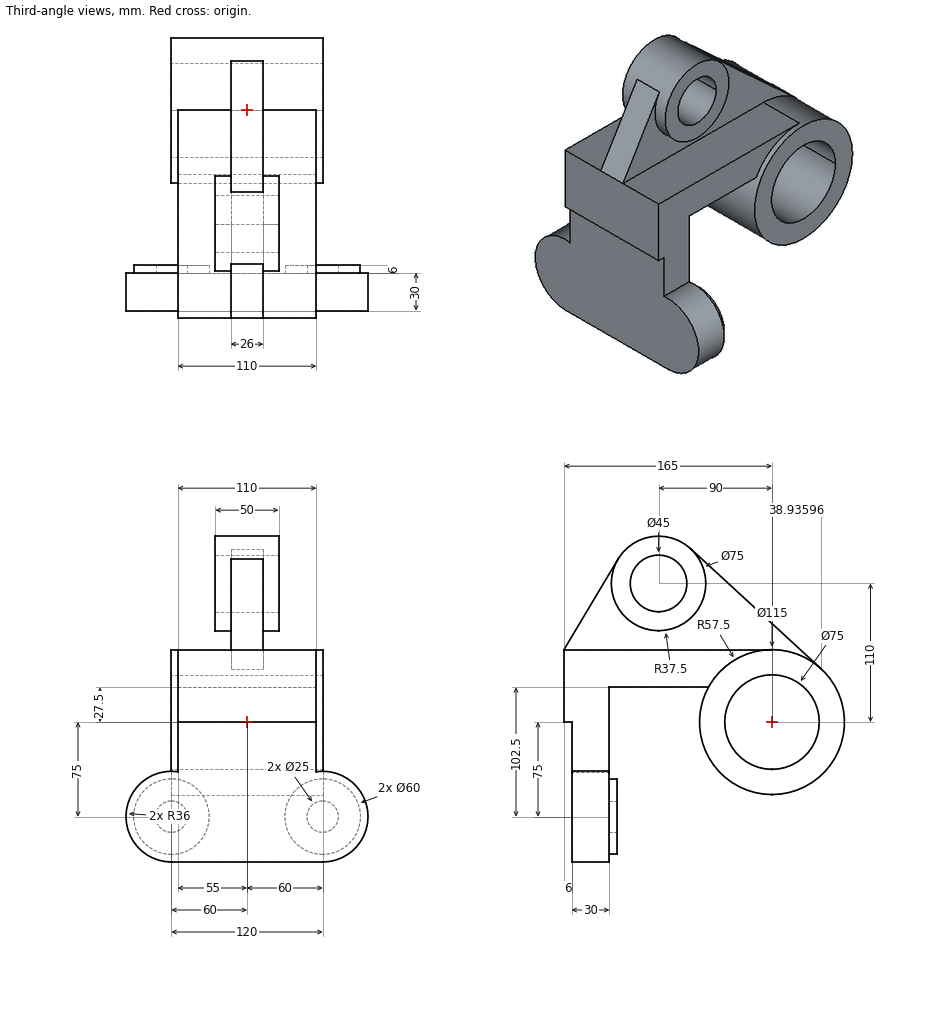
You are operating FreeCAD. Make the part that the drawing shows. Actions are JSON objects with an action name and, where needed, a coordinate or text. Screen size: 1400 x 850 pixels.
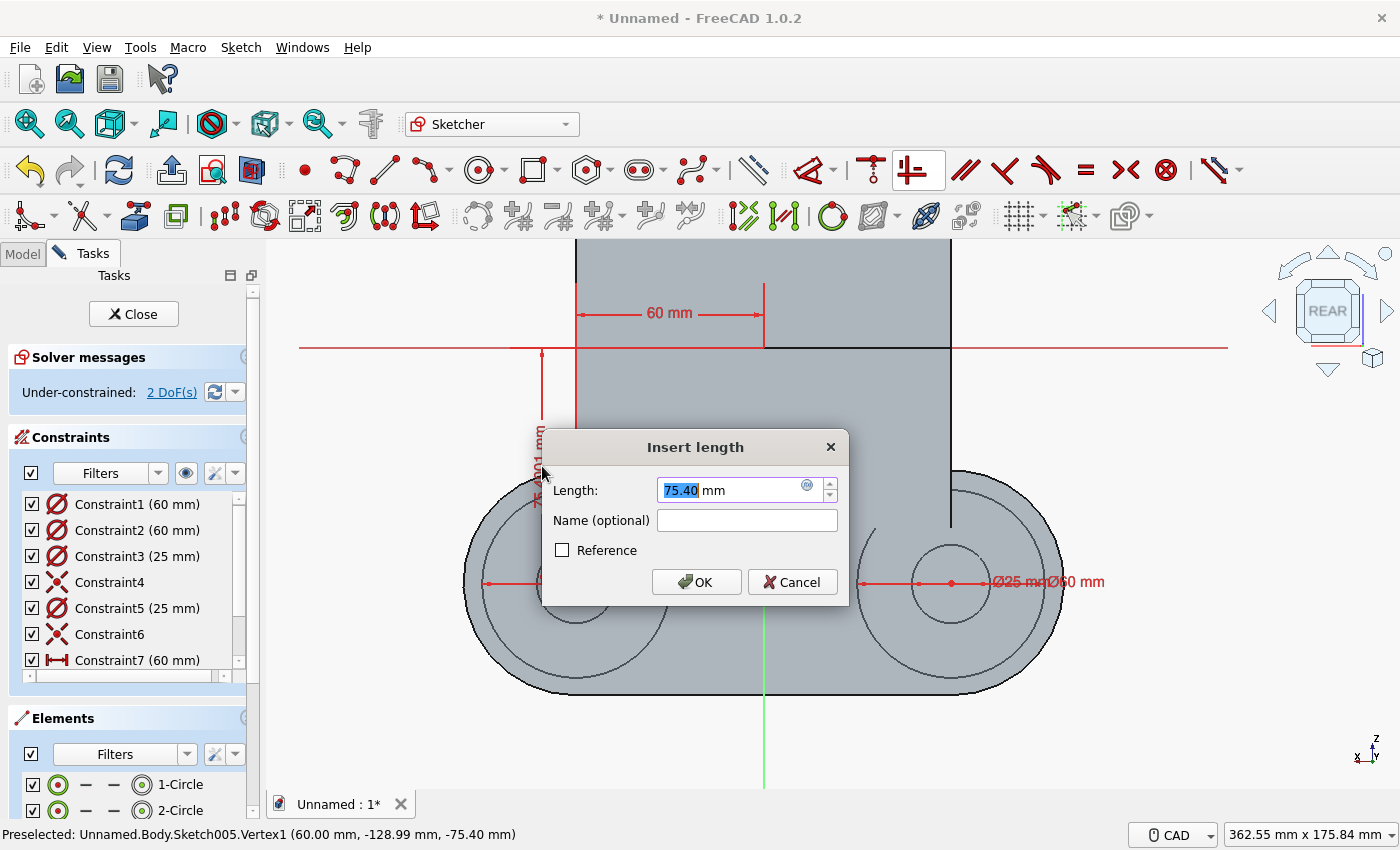
{"action": "type", "text": "75"}
{"action": "key", "text": "Return"}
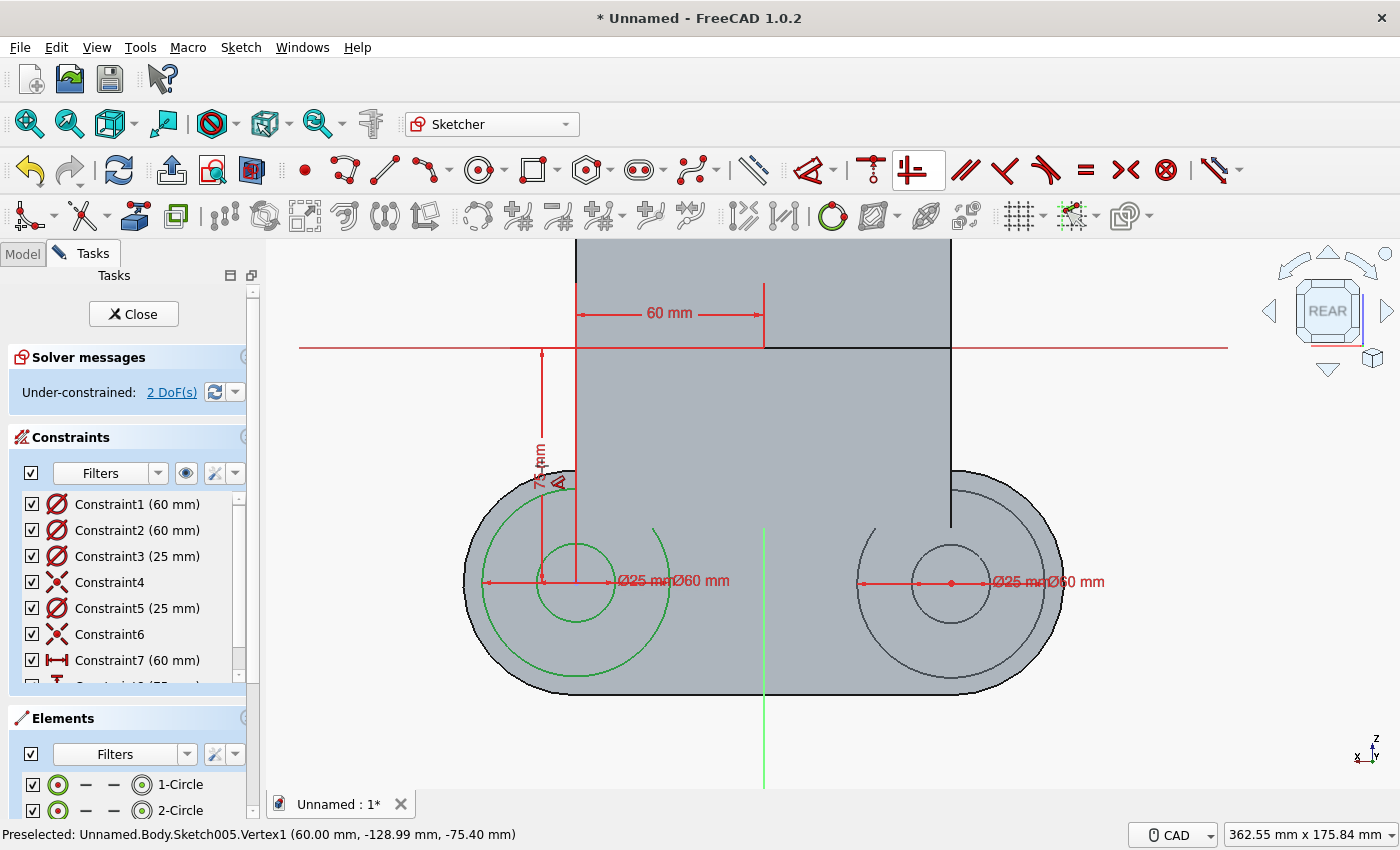
{"action": "left_click", "coordinate": [951, 584]}
{"action": "left_click", "coordinate": [857, 314]}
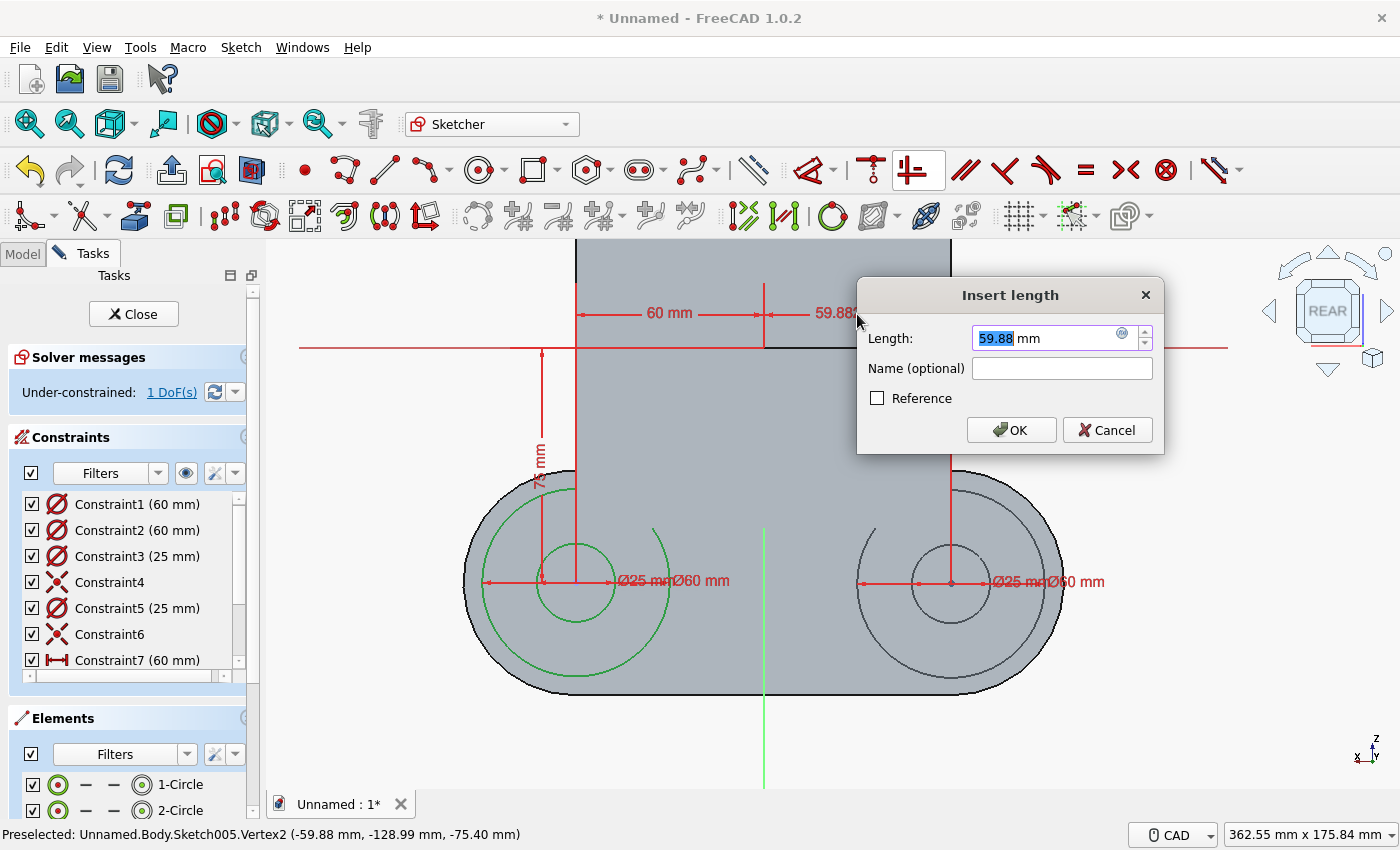
{"action": "type", "text": "60"}
{"action": "key", "text": "Return"}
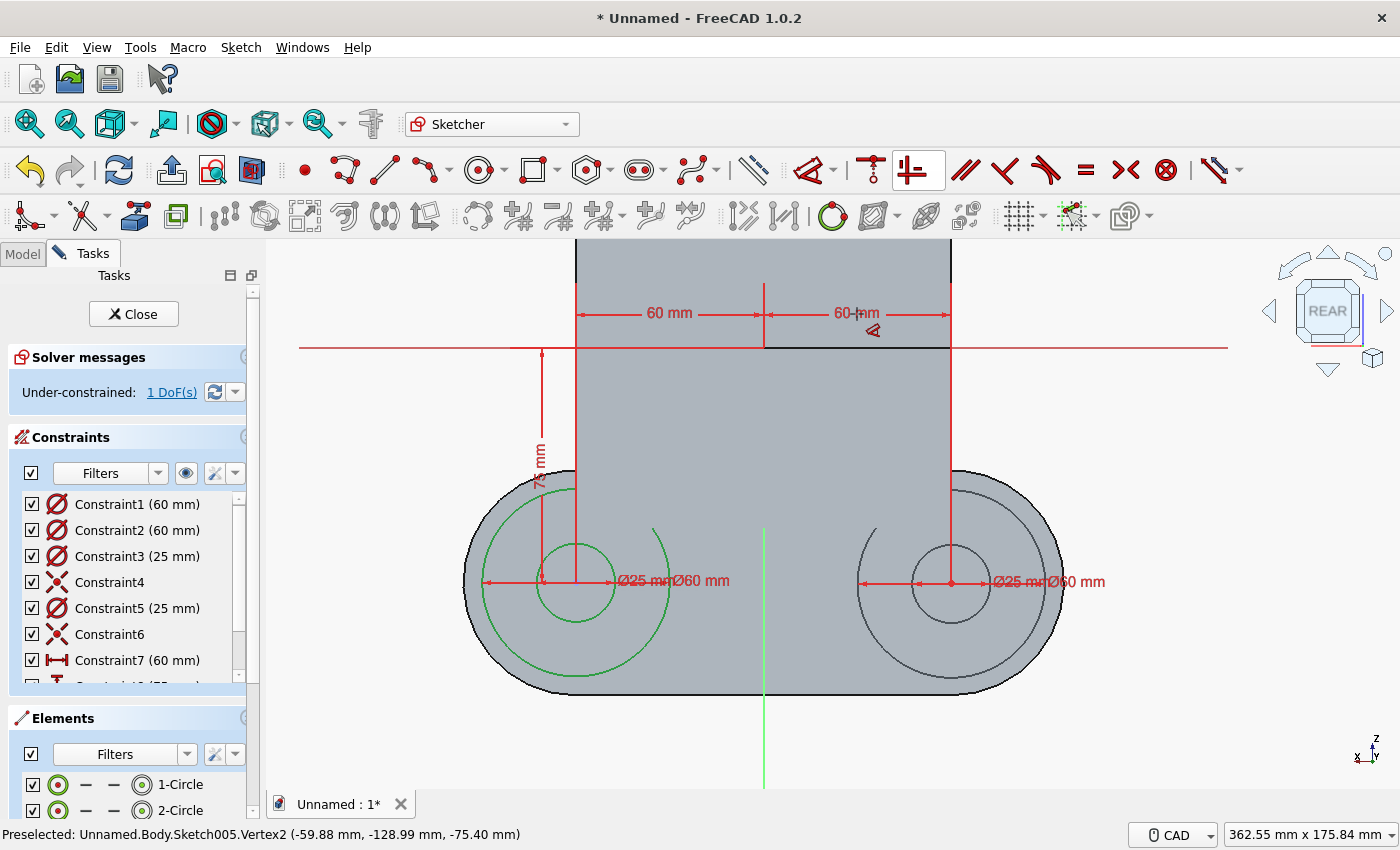
{"action": "left_click", "coordinate": [951, 584]}
{"action": "left_click", "coordinate": [985, 466]}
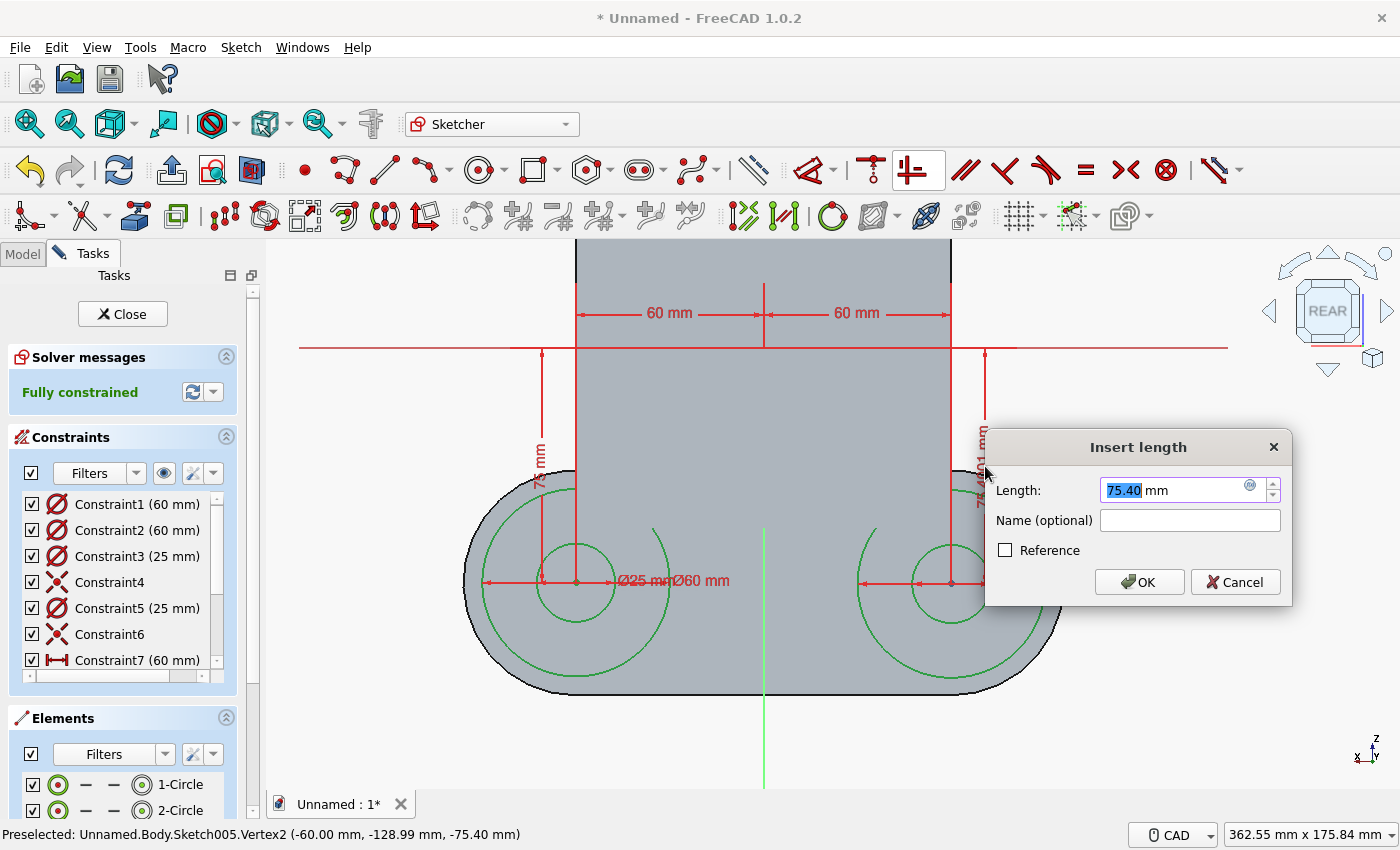
{"action": "type", "text": "75"}
{"action": "key", "text": "Return"}
{"action": "key", "text": "Escape"}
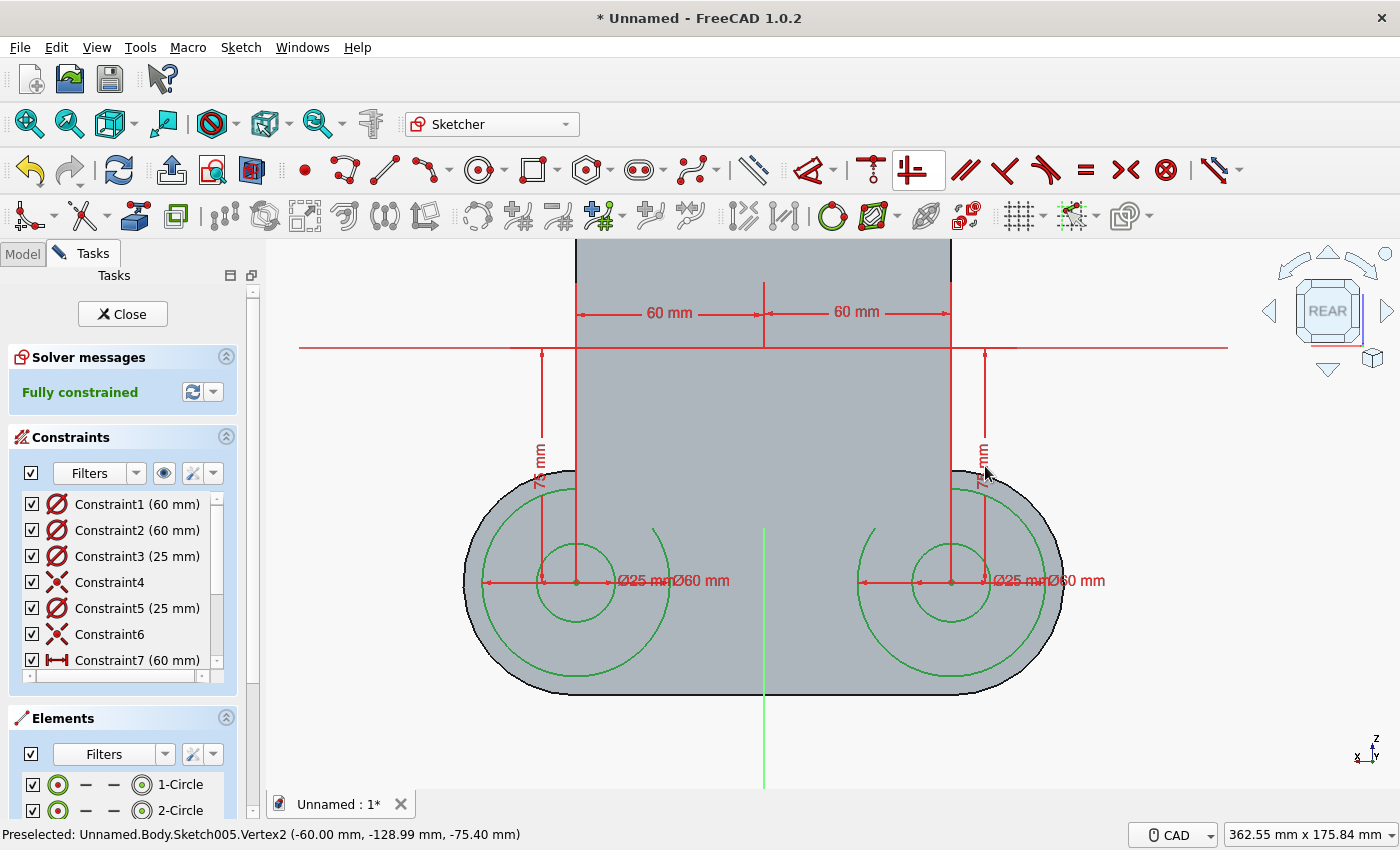
{"action": "left_click", "coordinate": [123, 314]}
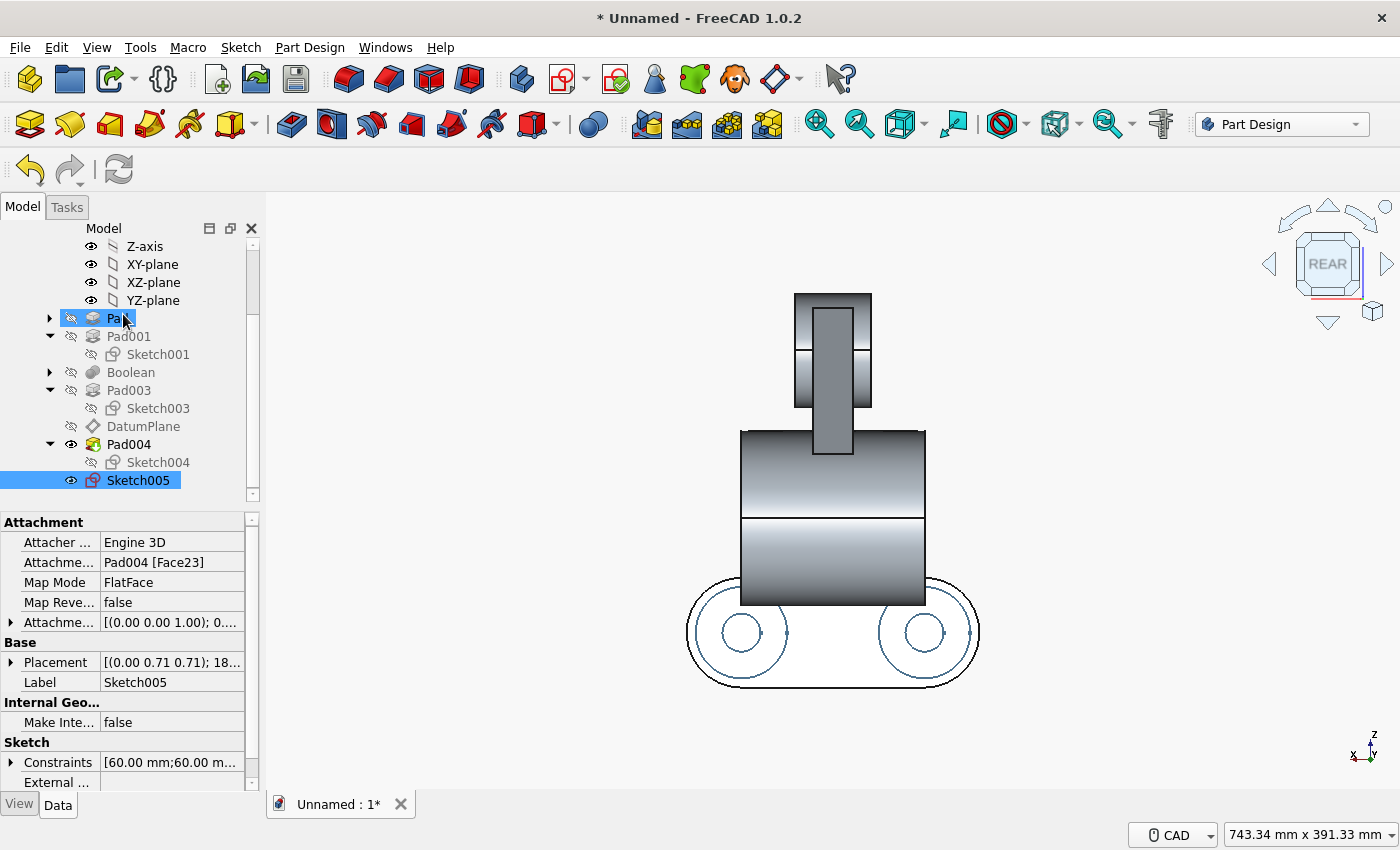
{"action": "left_click", "coordinate": [30, 124]}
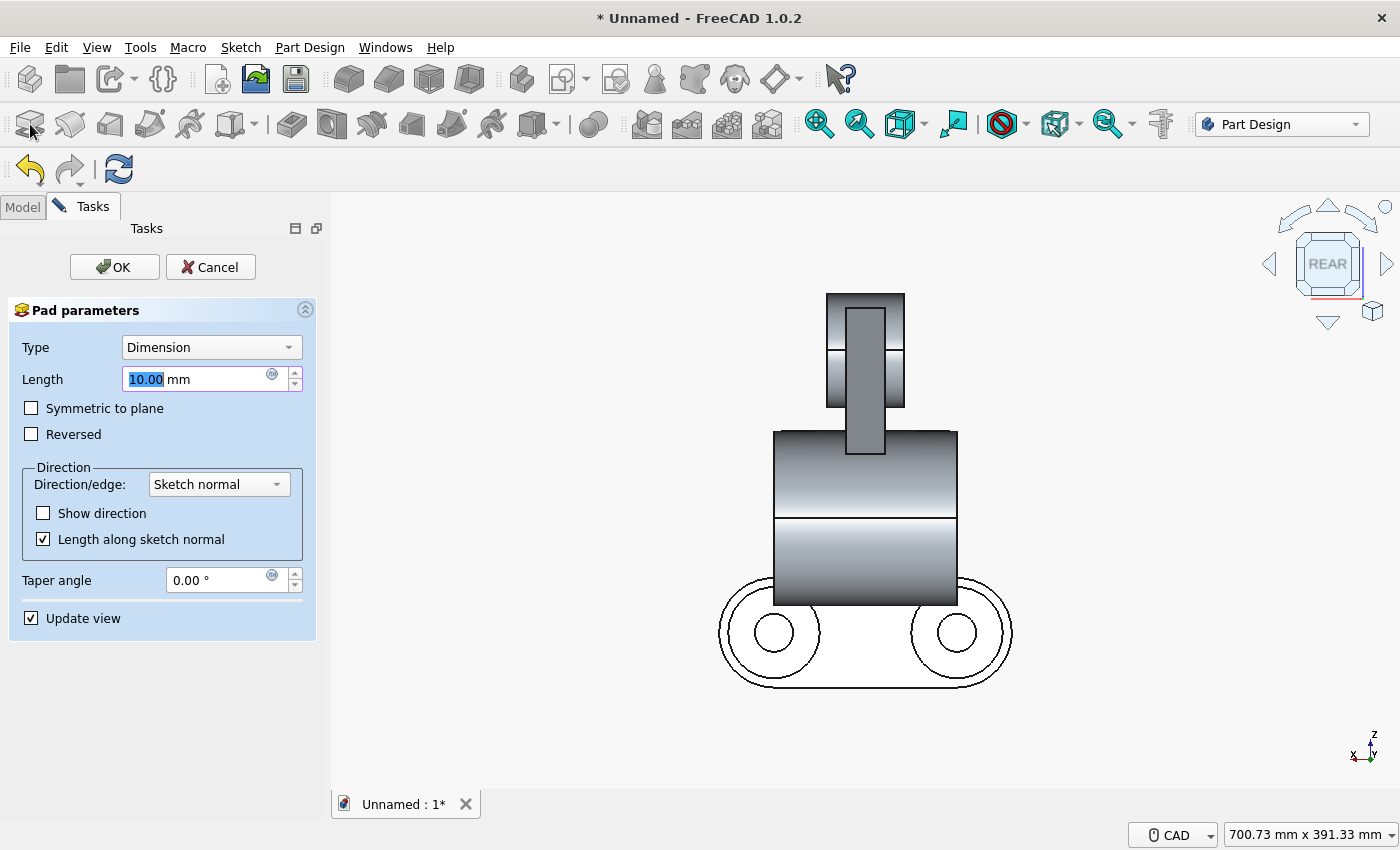
{"action": "type", "text": "6"}
{"action": "key", "text": "Tab"}